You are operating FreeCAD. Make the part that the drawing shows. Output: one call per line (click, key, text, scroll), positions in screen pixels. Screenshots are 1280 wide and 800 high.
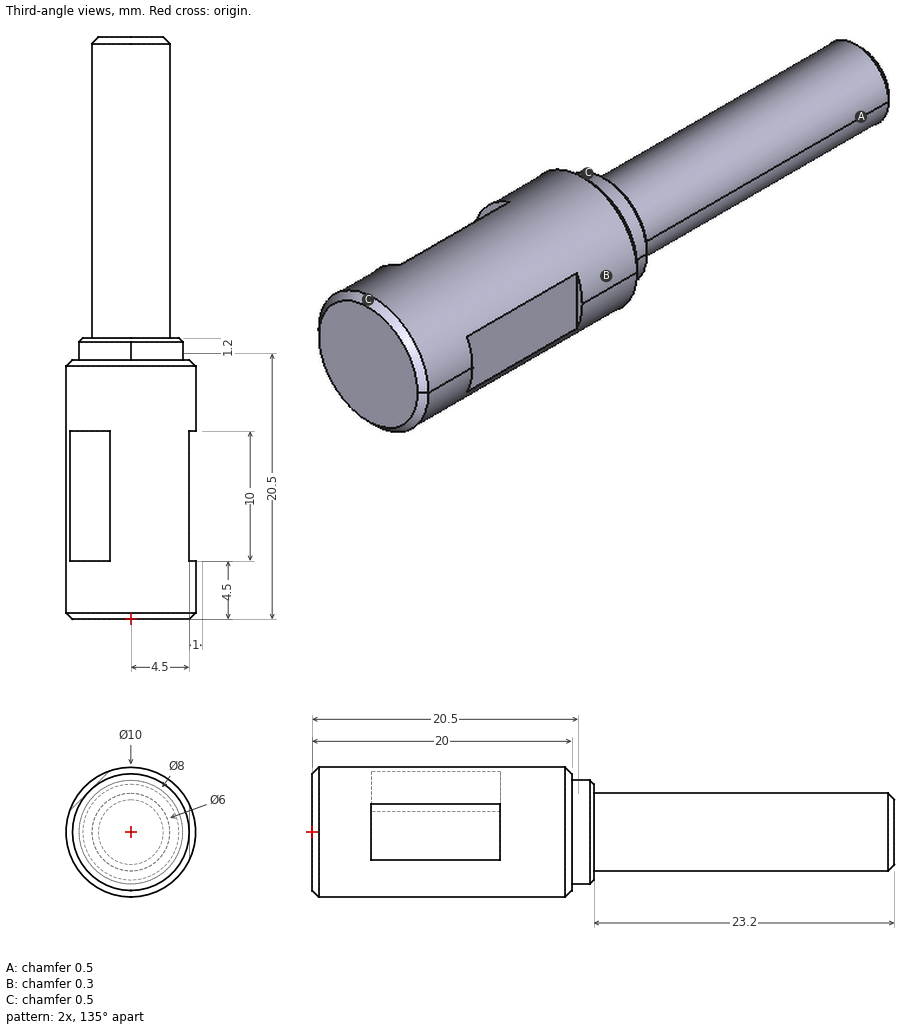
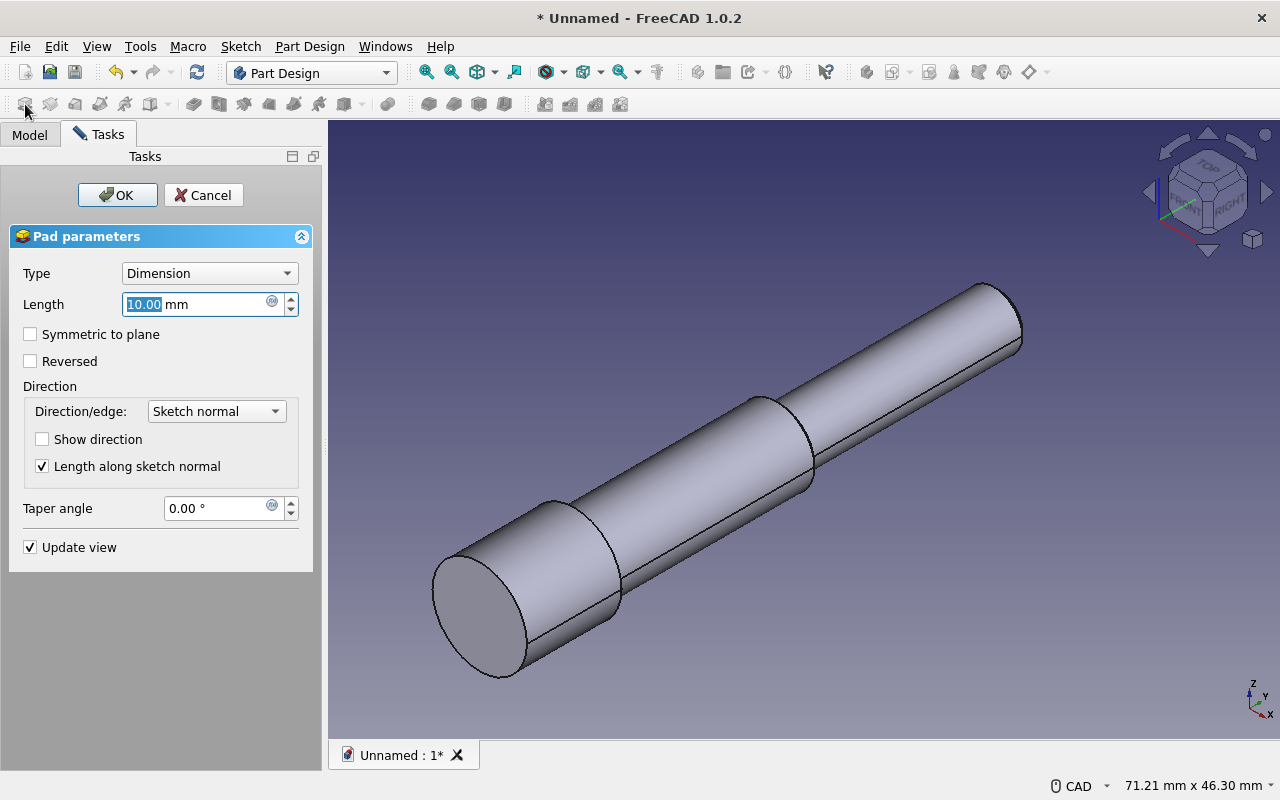
text(20)
key(Tab)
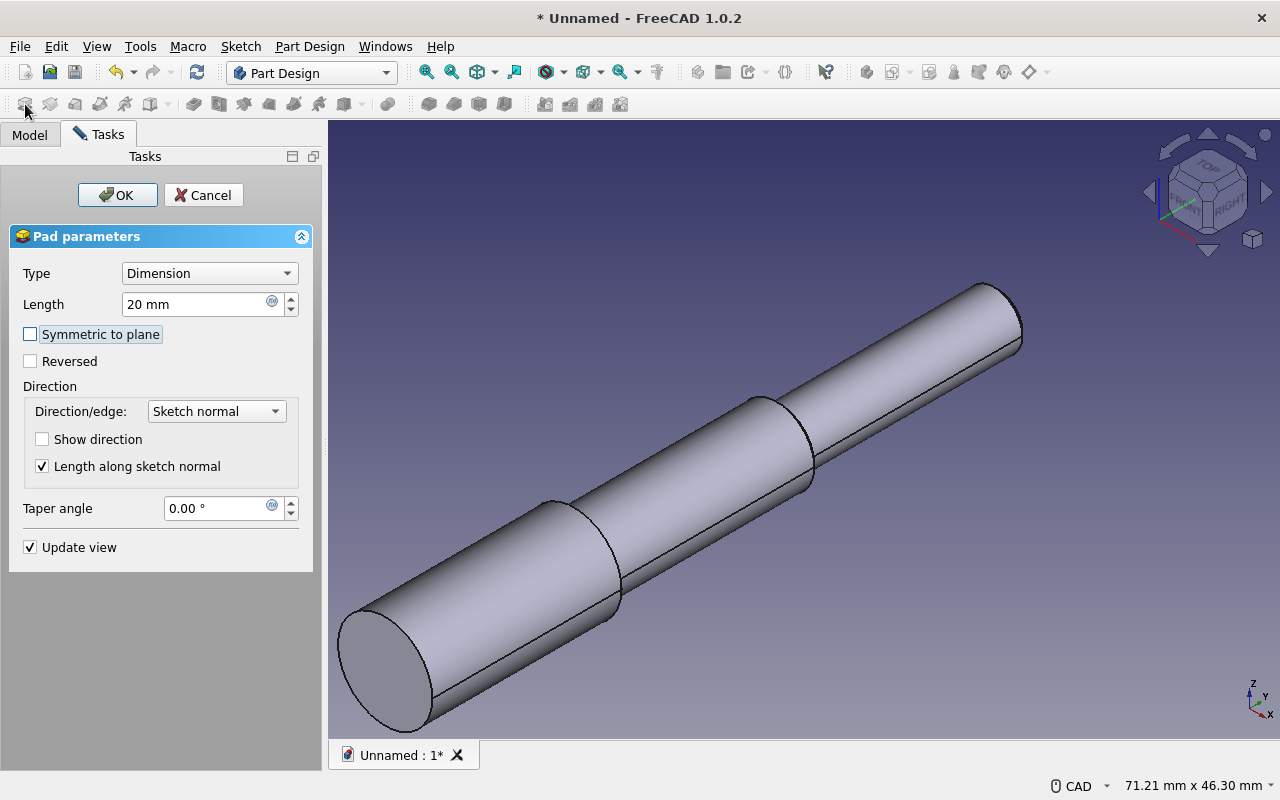
click(31, 361)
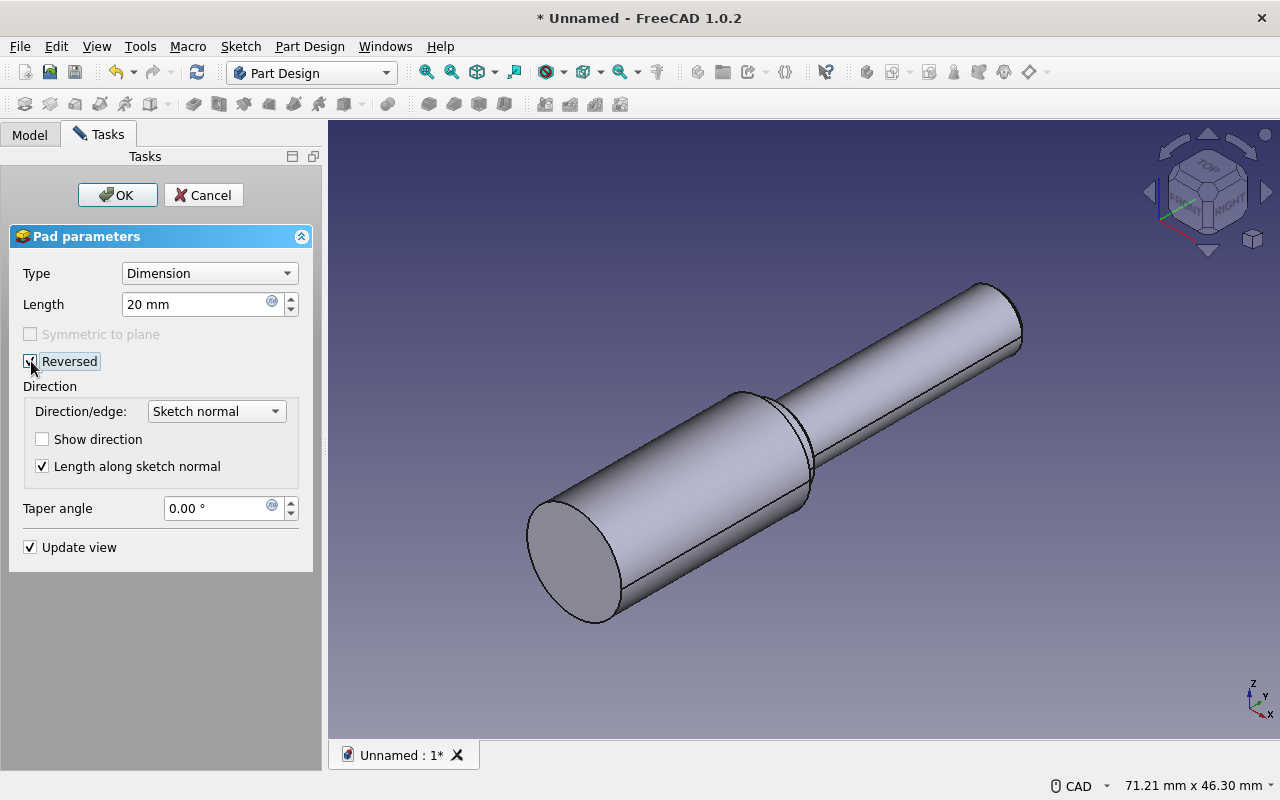
click(118, 195)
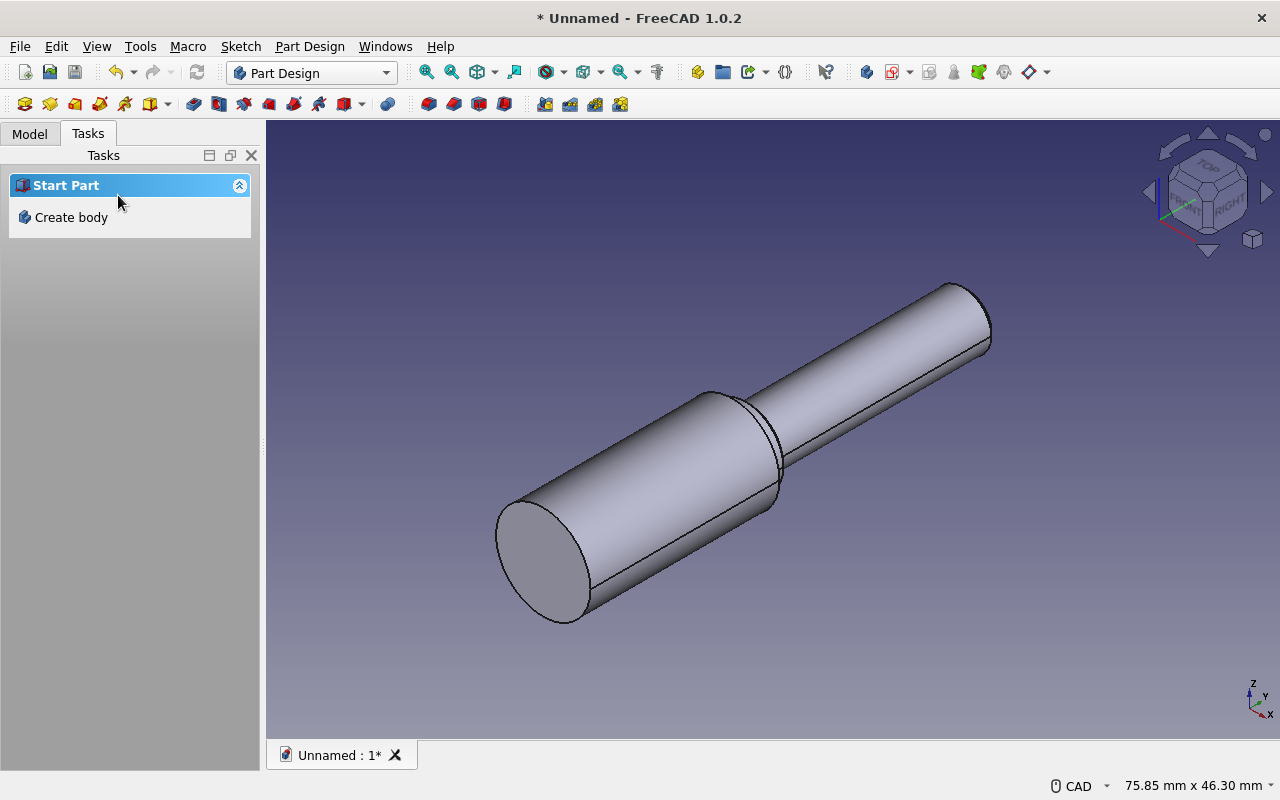
click(529, 501)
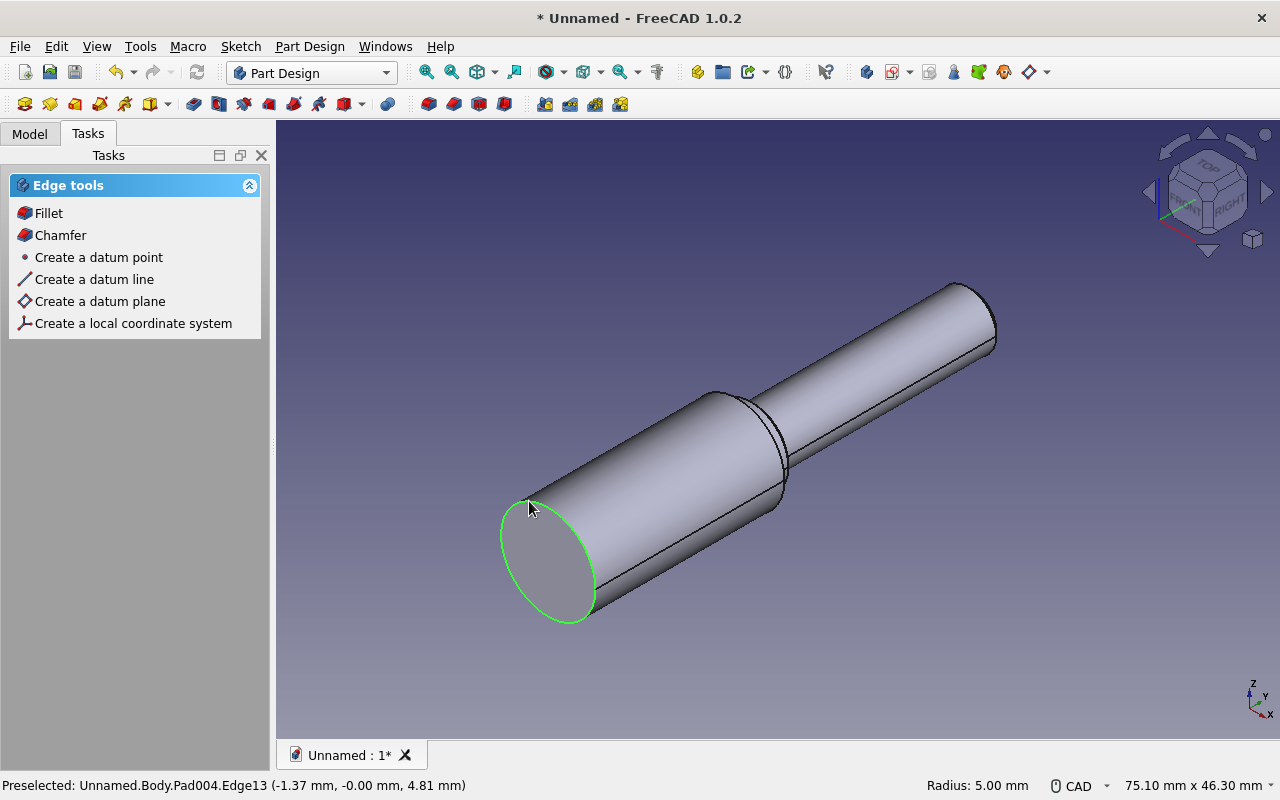
key(2)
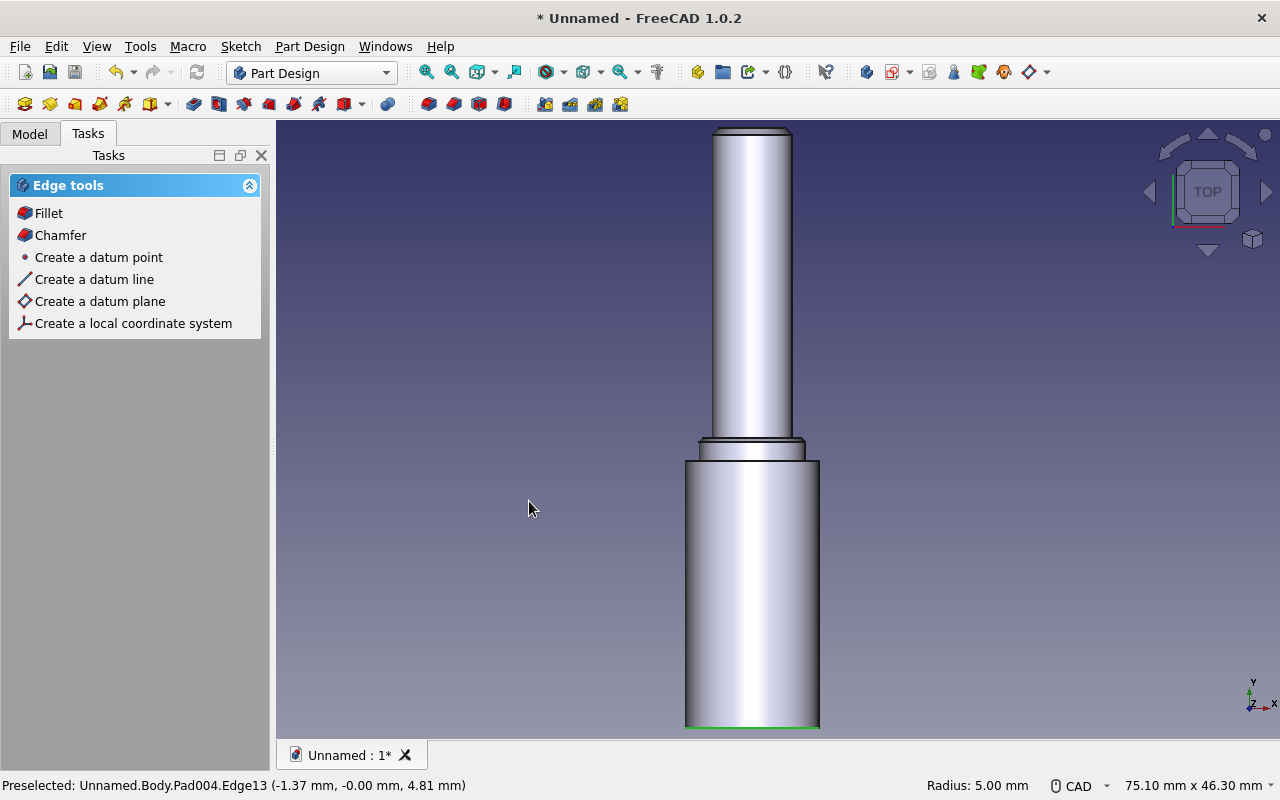
click(698, 460, ctrl)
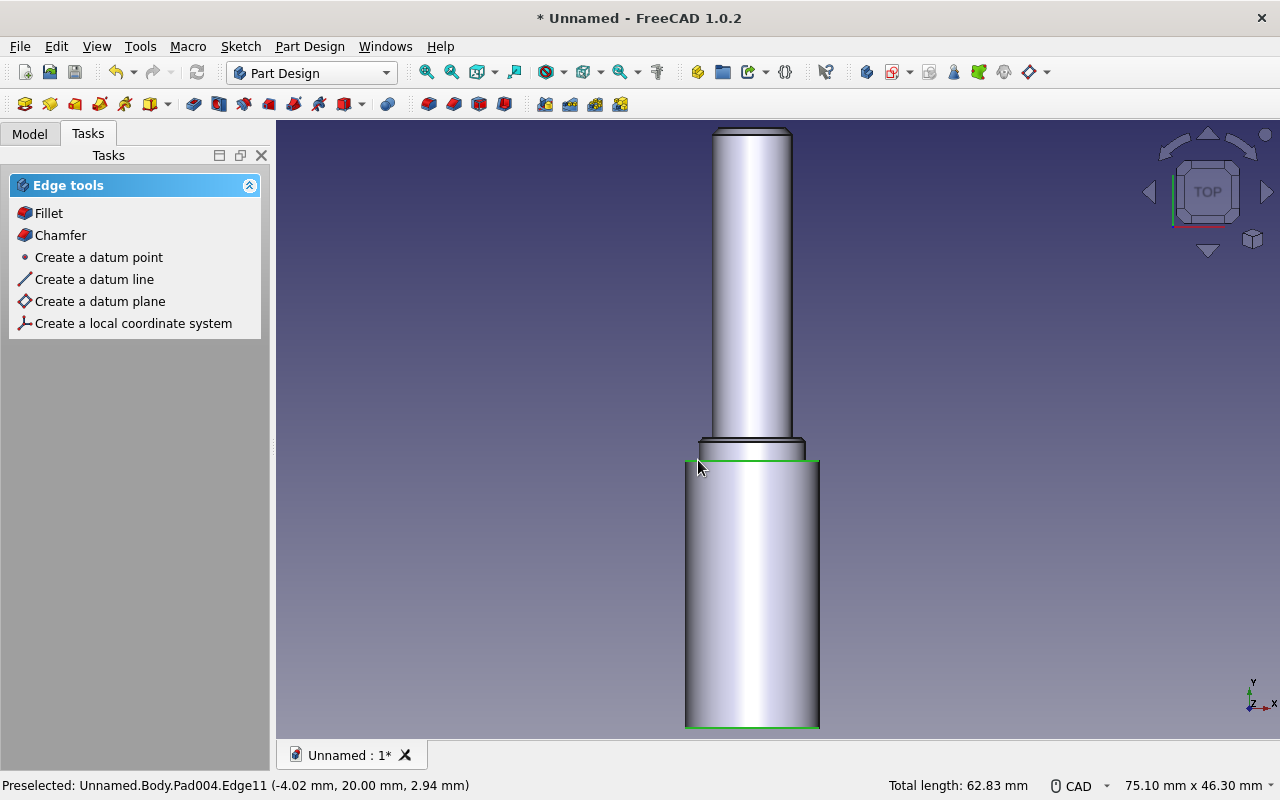
click(454, 104)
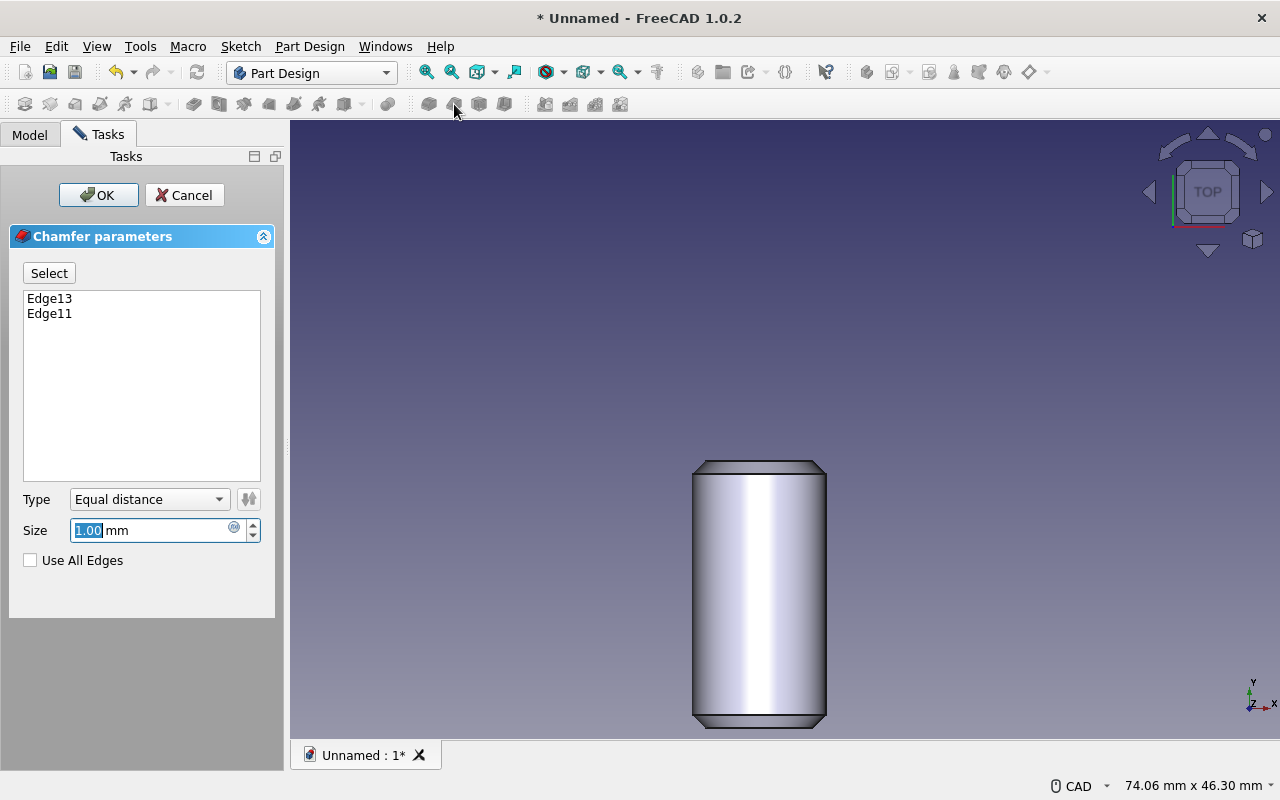
text(0.5)
key(Tab)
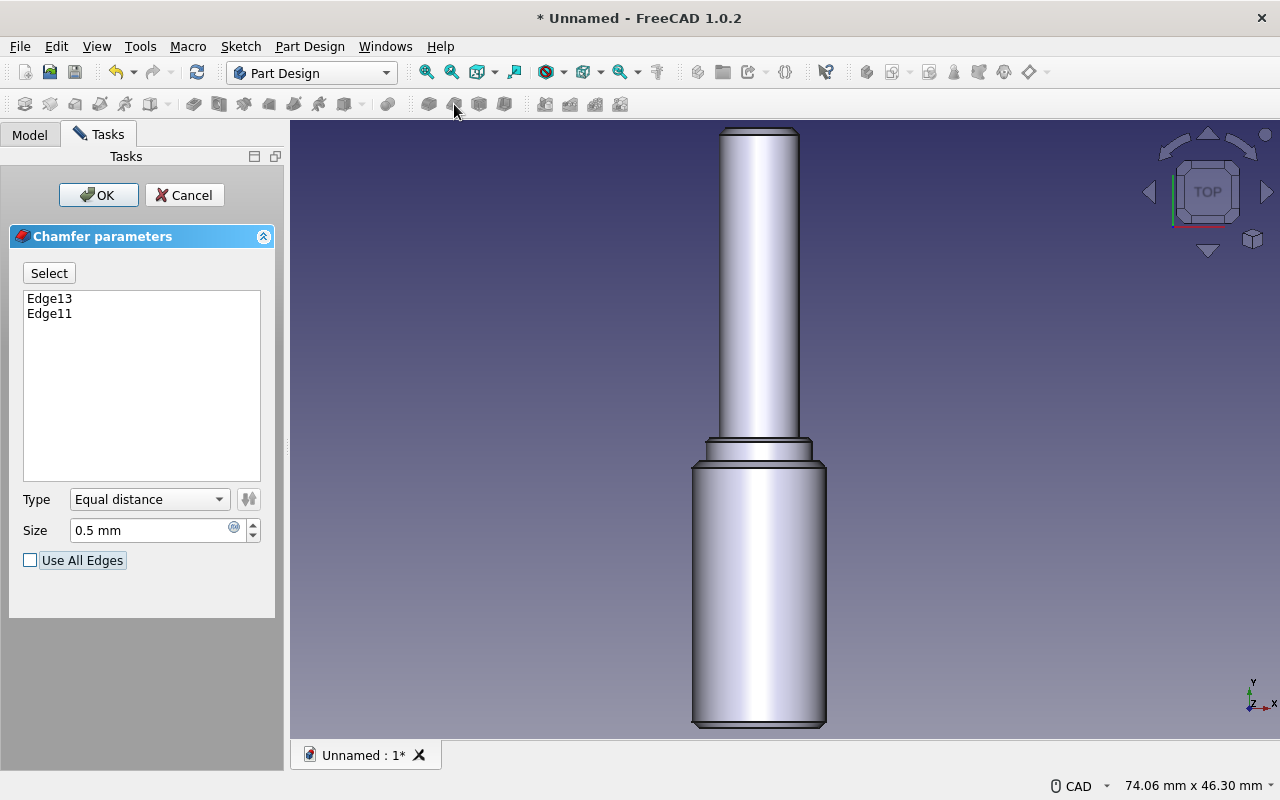
click(99, 195)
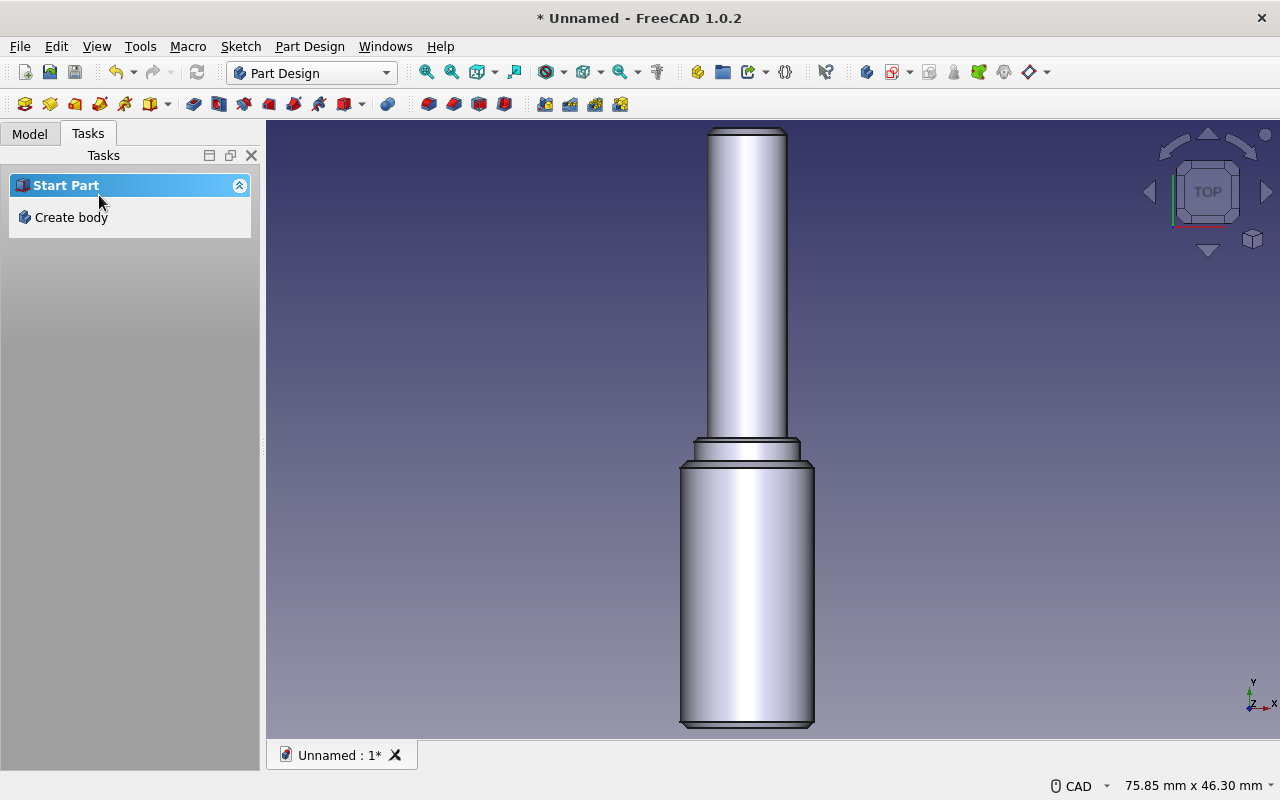
click(892, 72)